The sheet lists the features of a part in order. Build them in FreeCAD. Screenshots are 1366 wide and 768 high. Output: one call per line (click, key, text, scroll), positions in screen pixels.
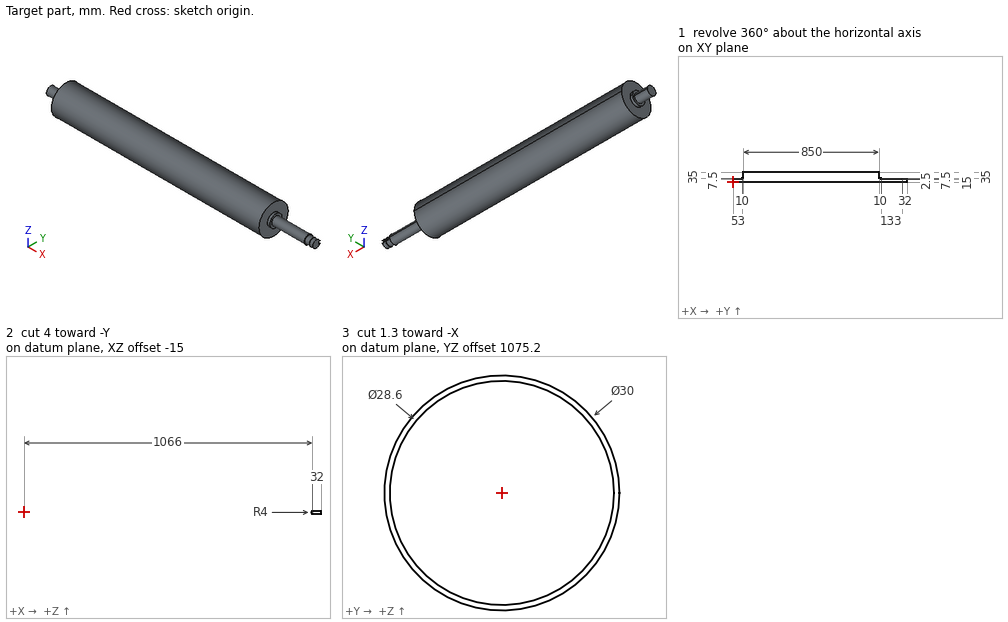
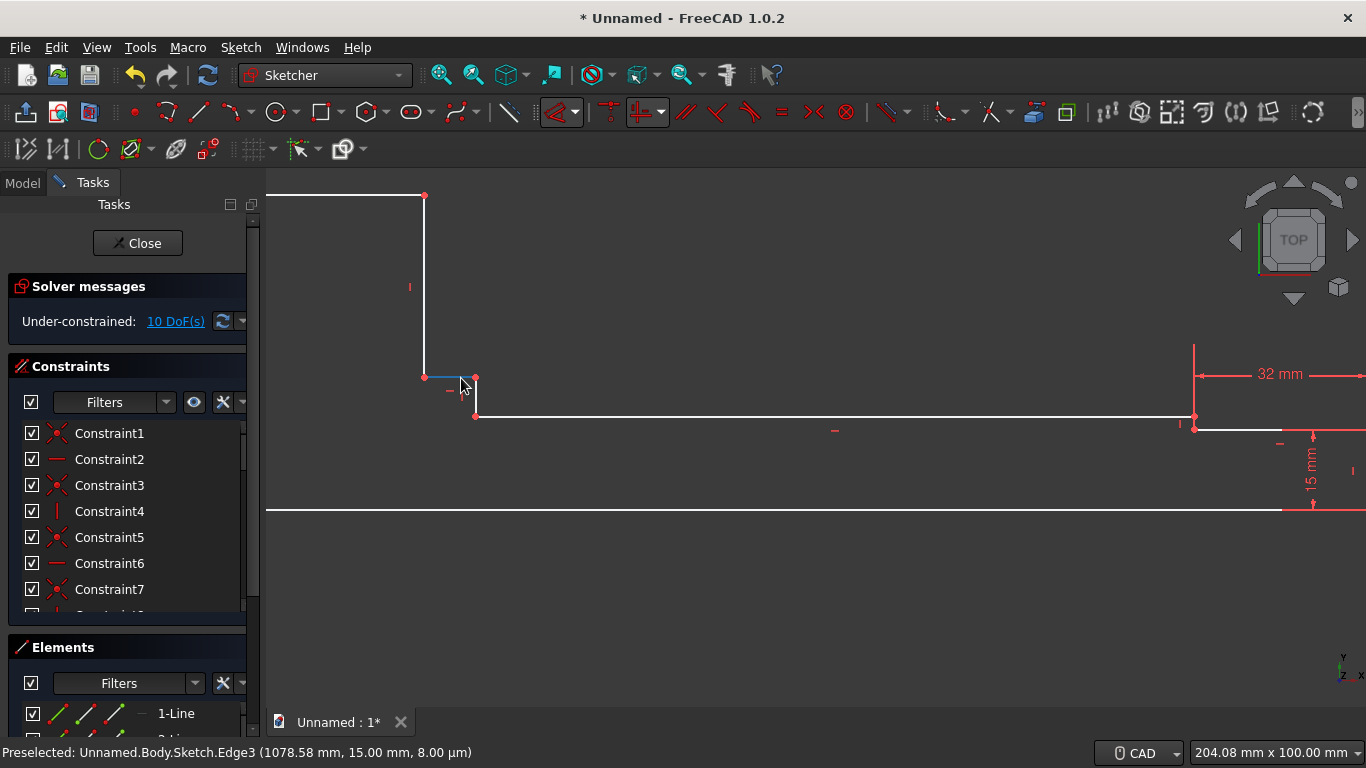
click(460, 377)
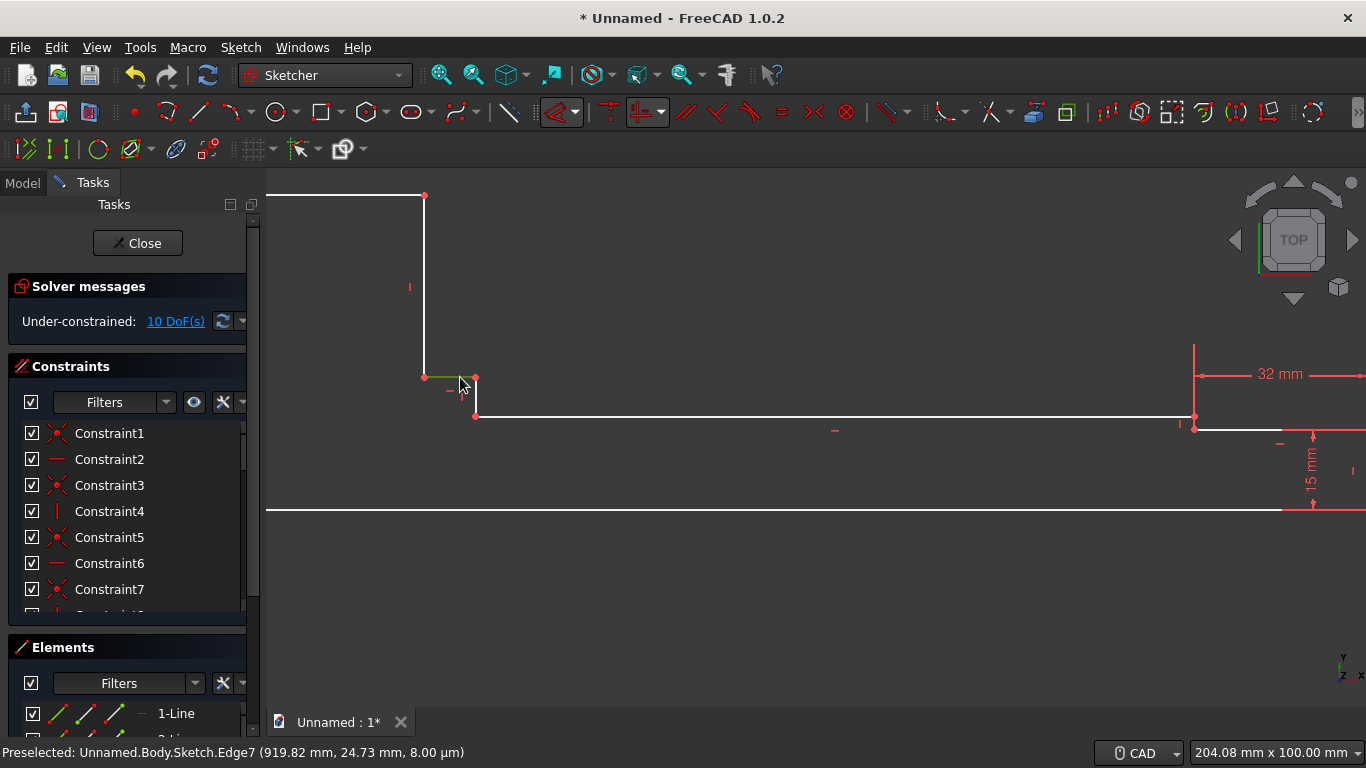
key(l)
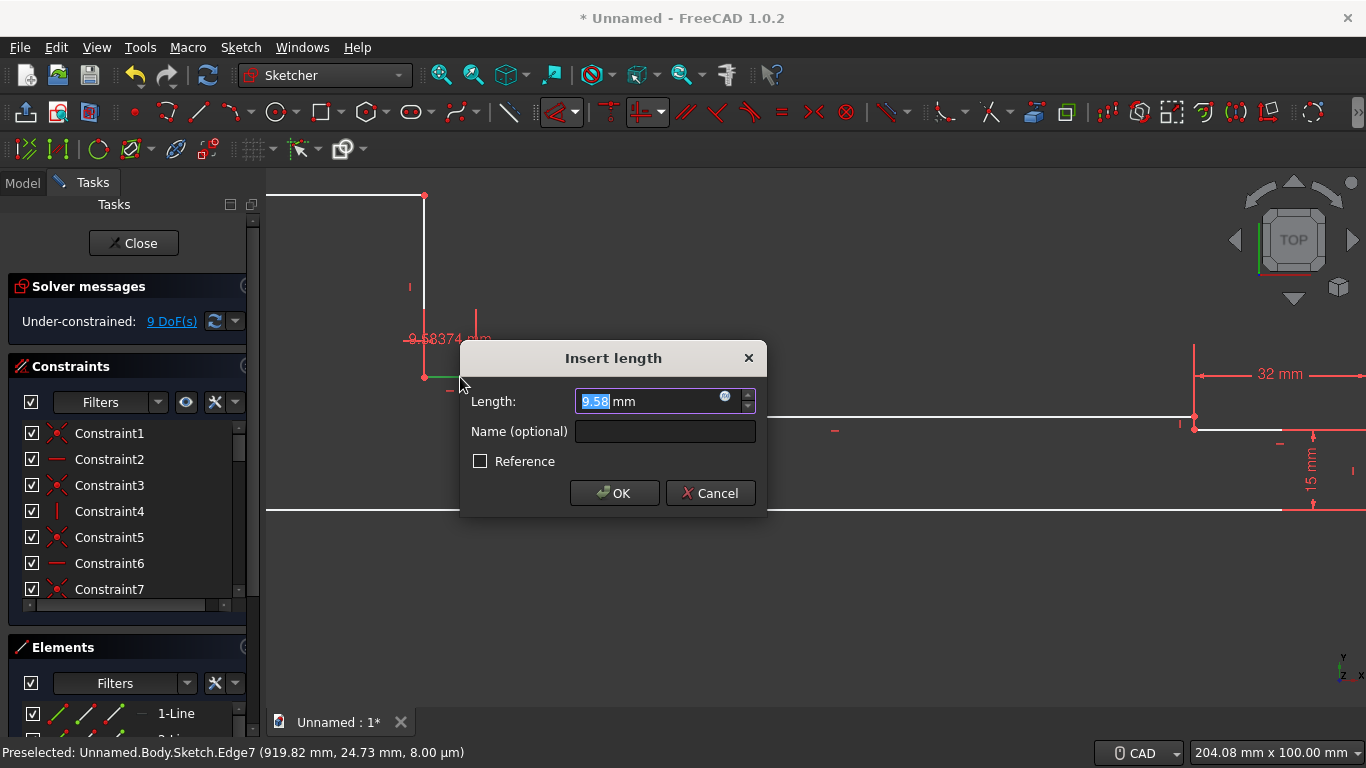
text(10)
key(Return)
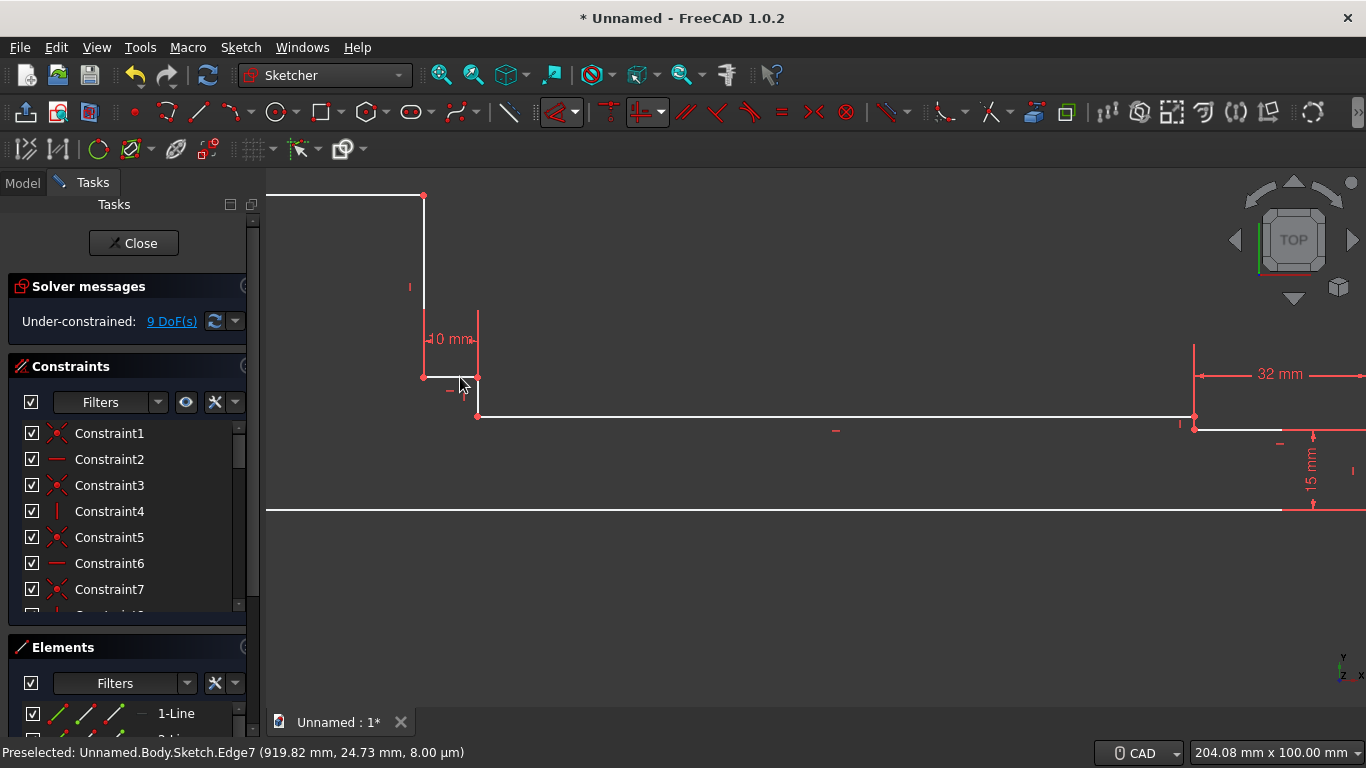
scroll(1036, 449, down, 11)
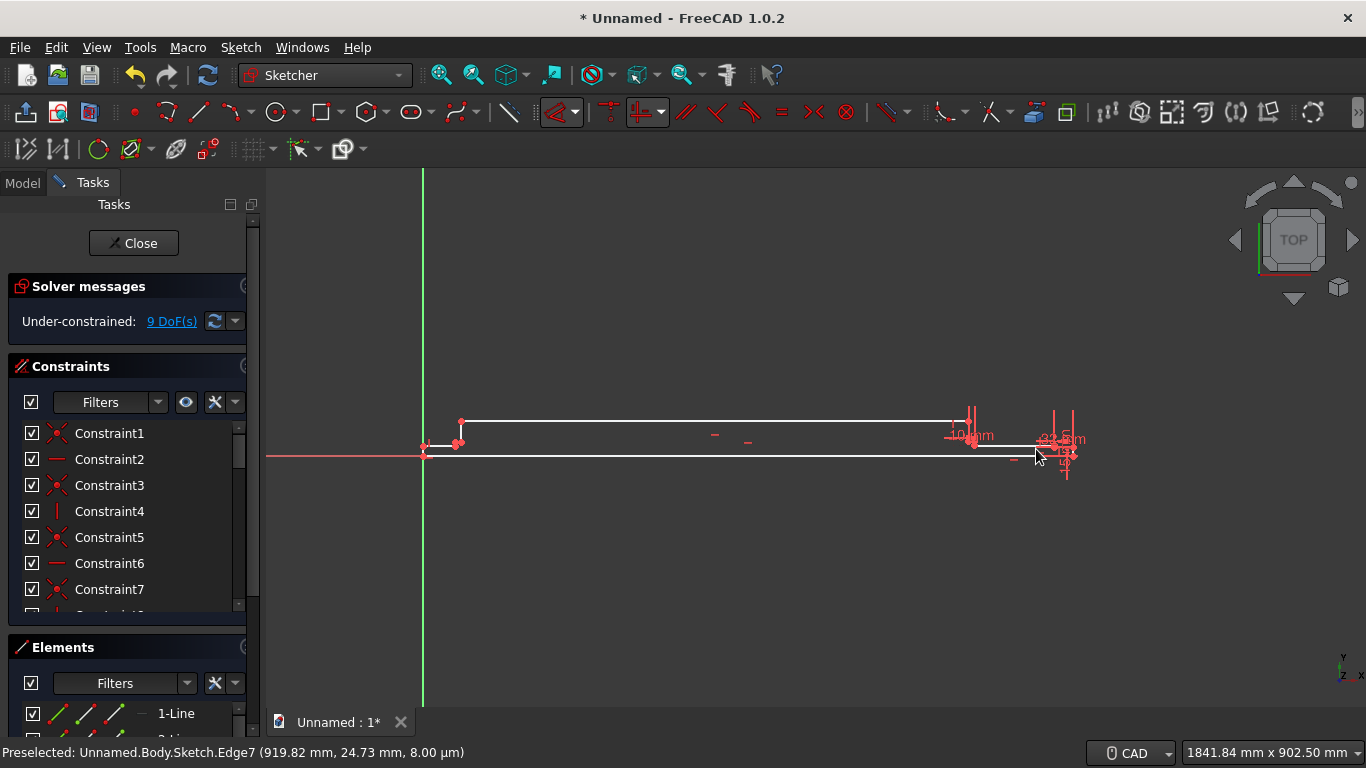
scroll(969, 435, up, 5)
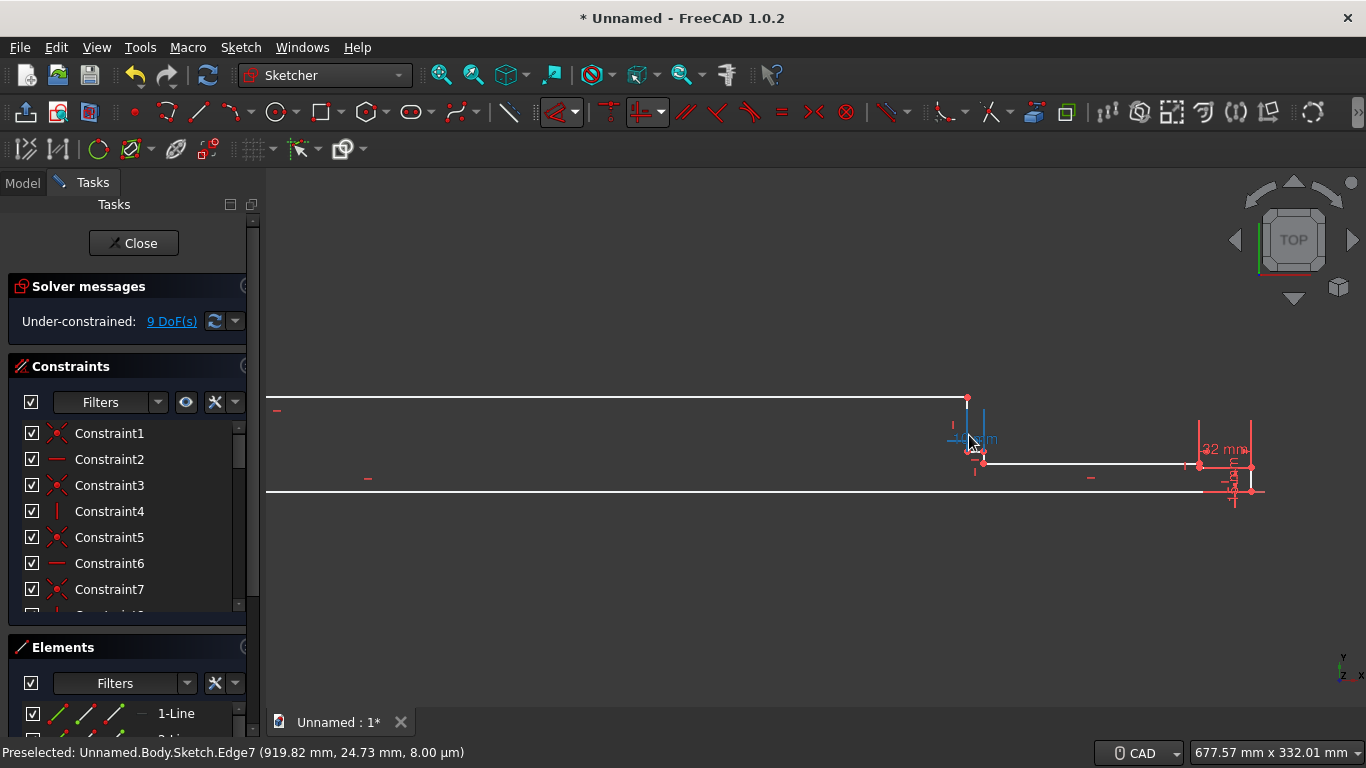
click(967, 413)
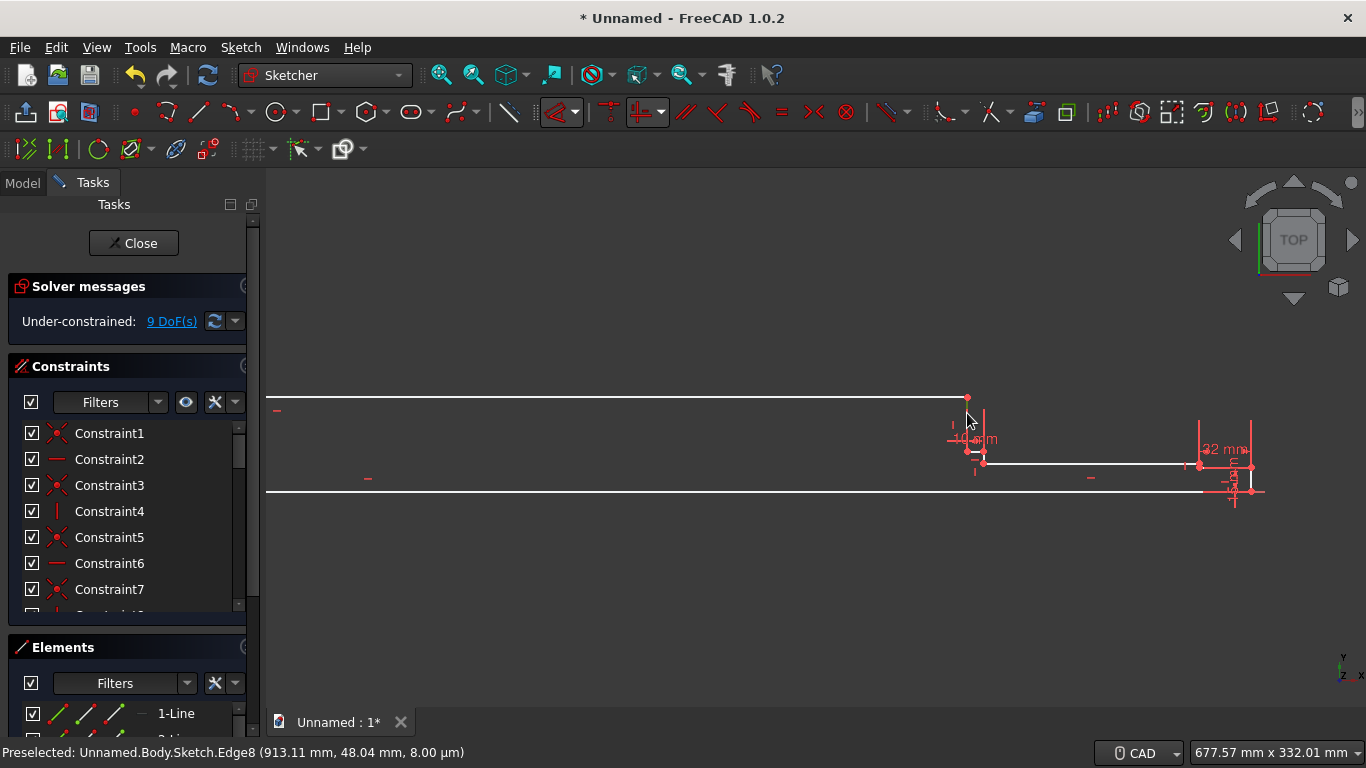
click(578, 112)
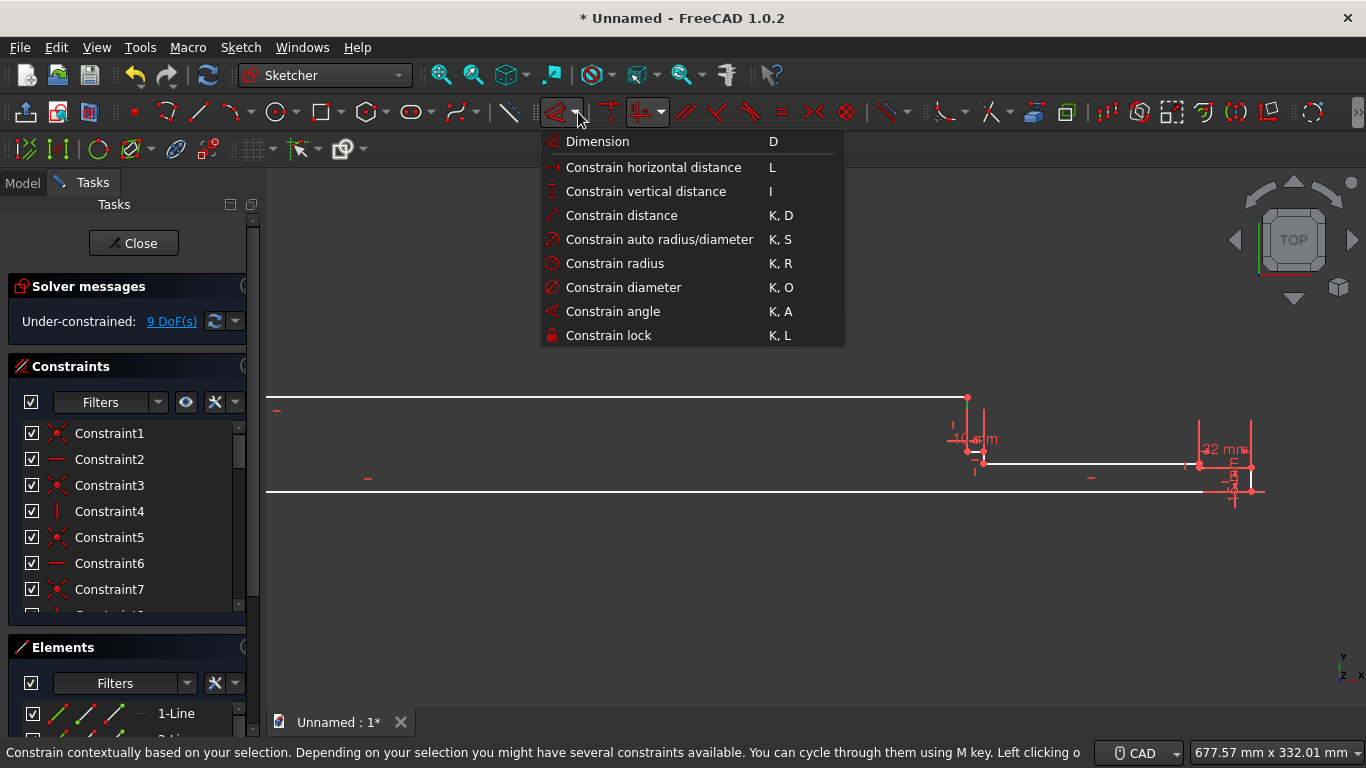
click(693, 191)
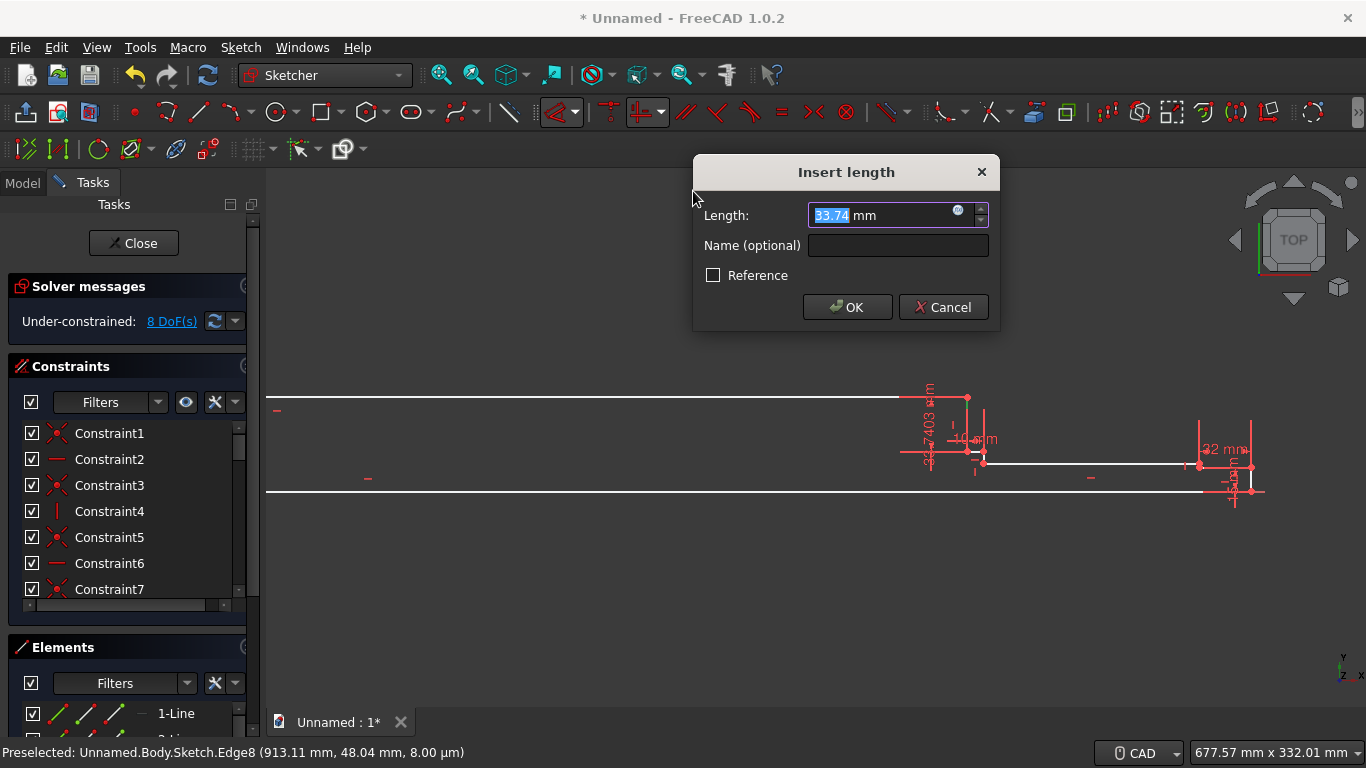
text(35)
key(Return)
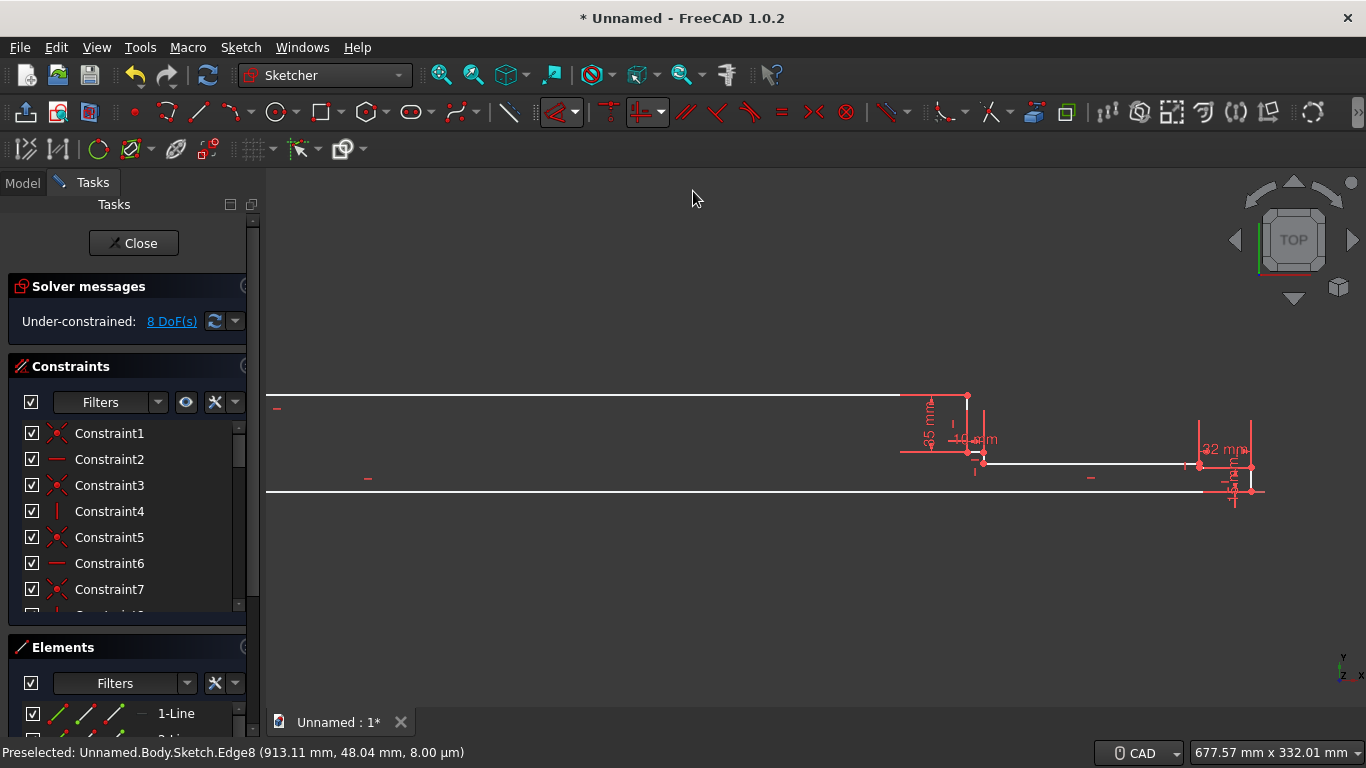
scroll(968, 434, down, 5)